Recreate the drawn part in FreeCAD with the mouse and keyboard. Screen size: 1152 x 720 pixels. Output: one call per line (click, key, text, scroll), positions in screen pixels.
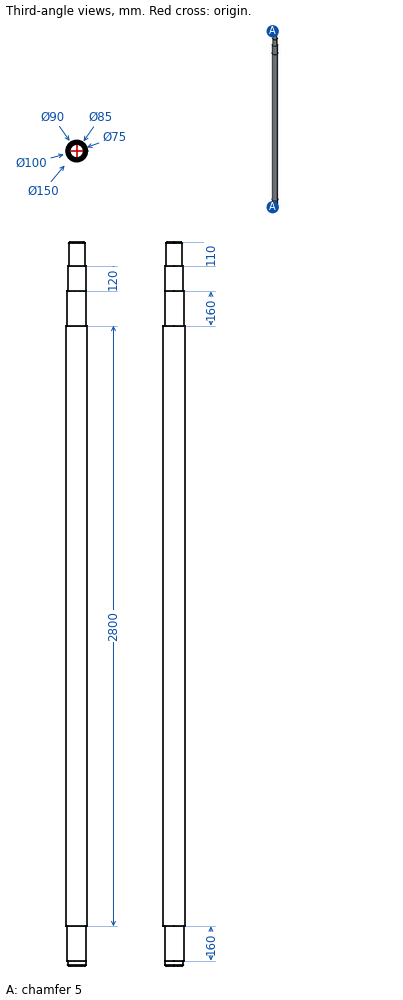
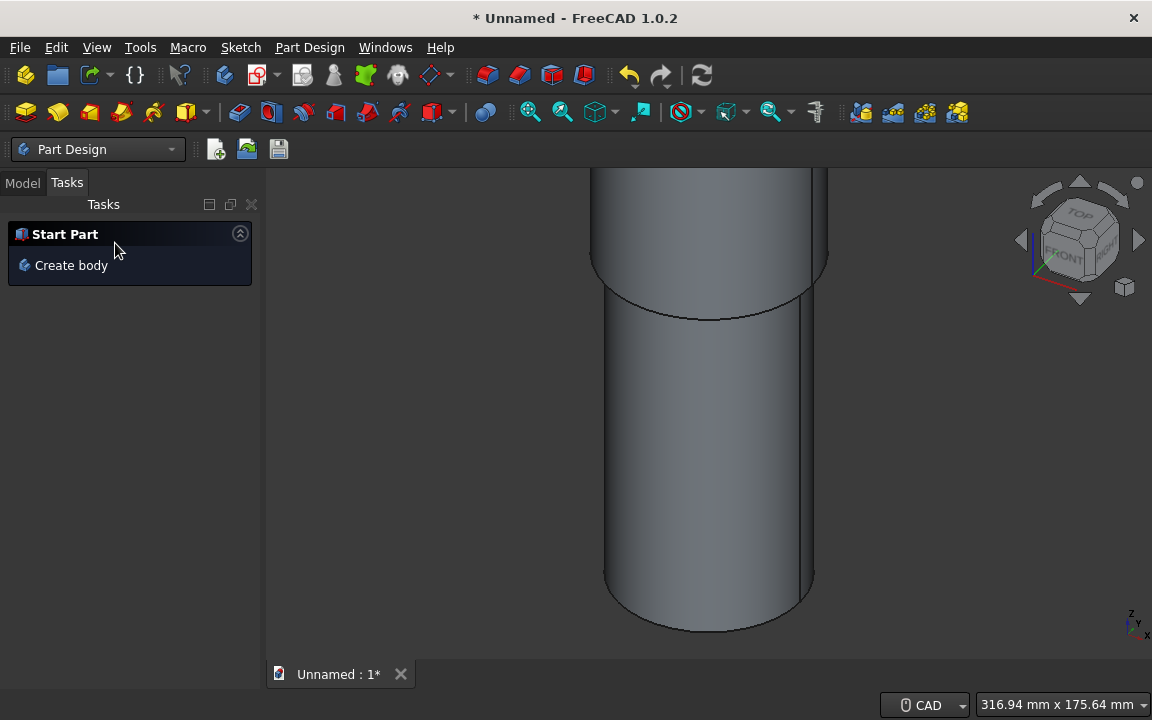
click(532, 112)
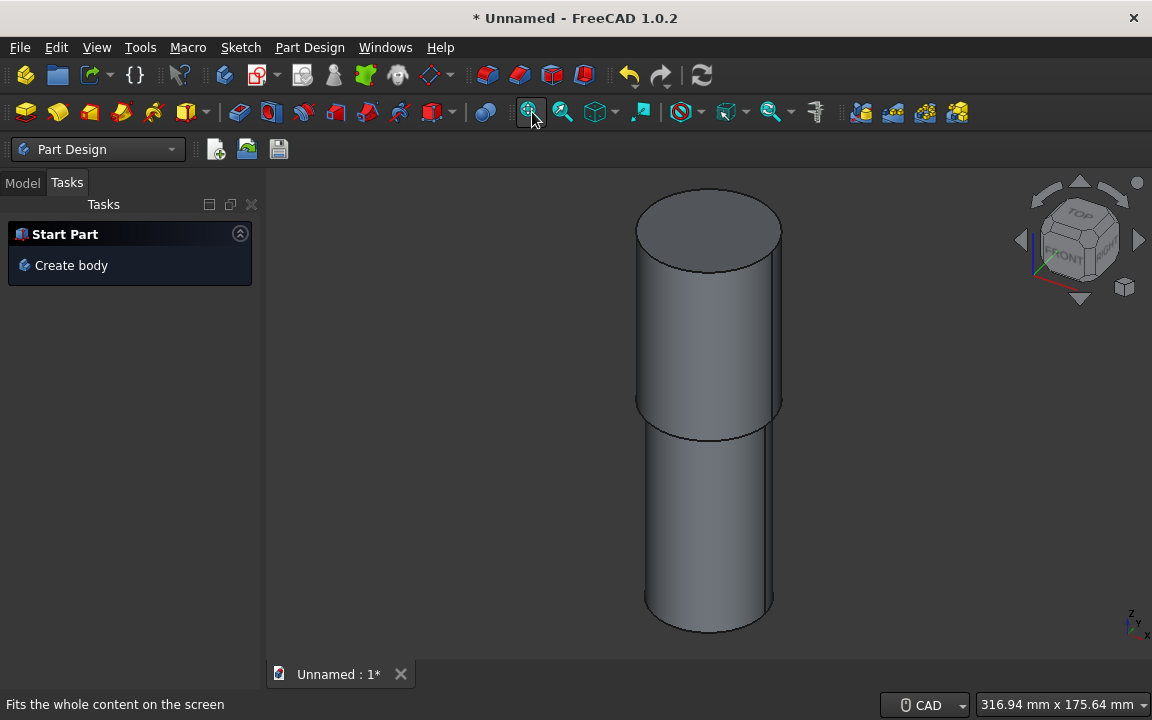
click(709, 230)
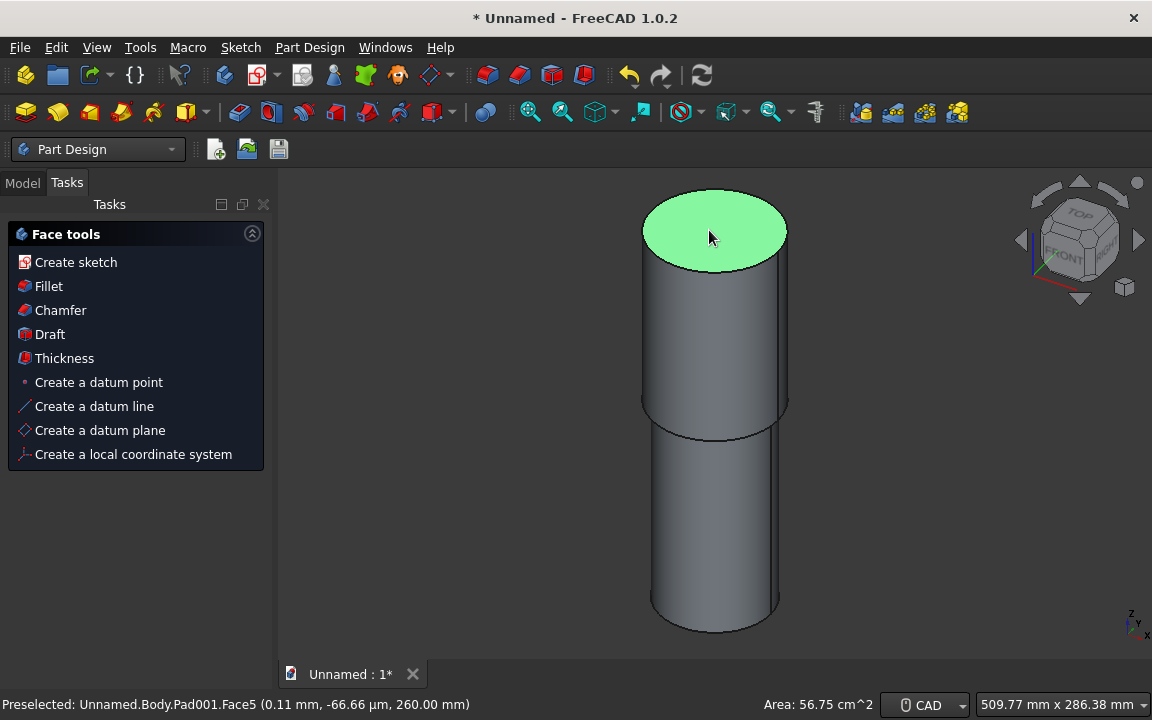
click(258, 76)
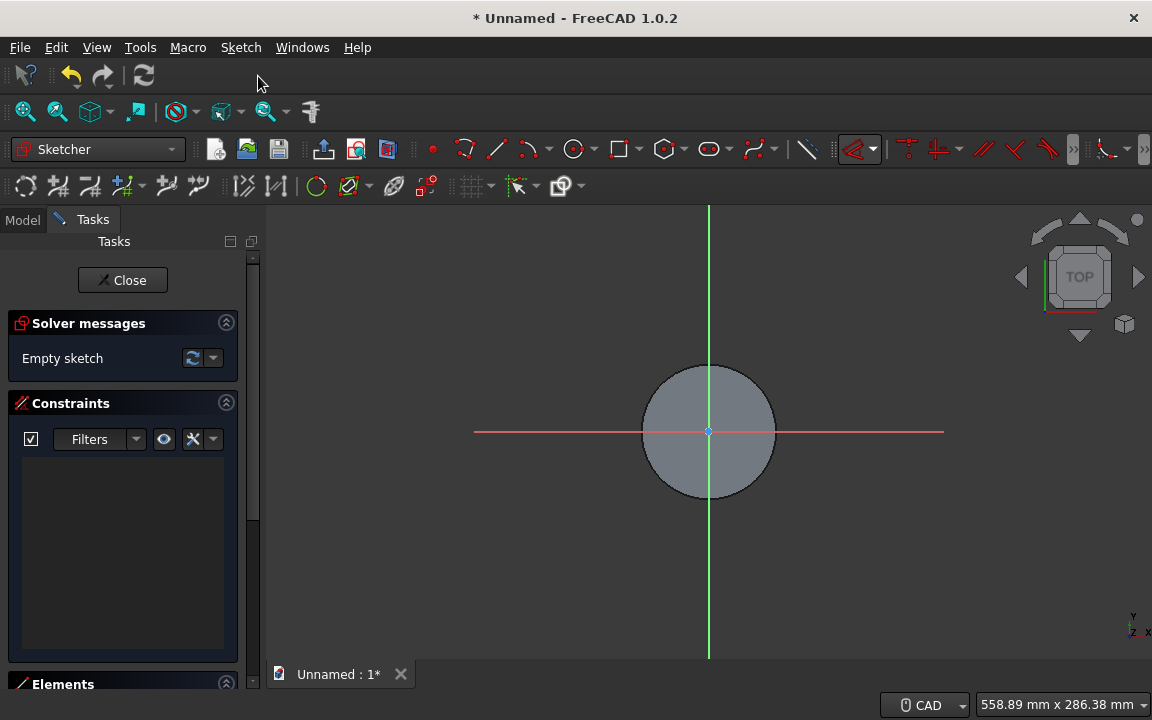
scroll(792, 432, up, 3)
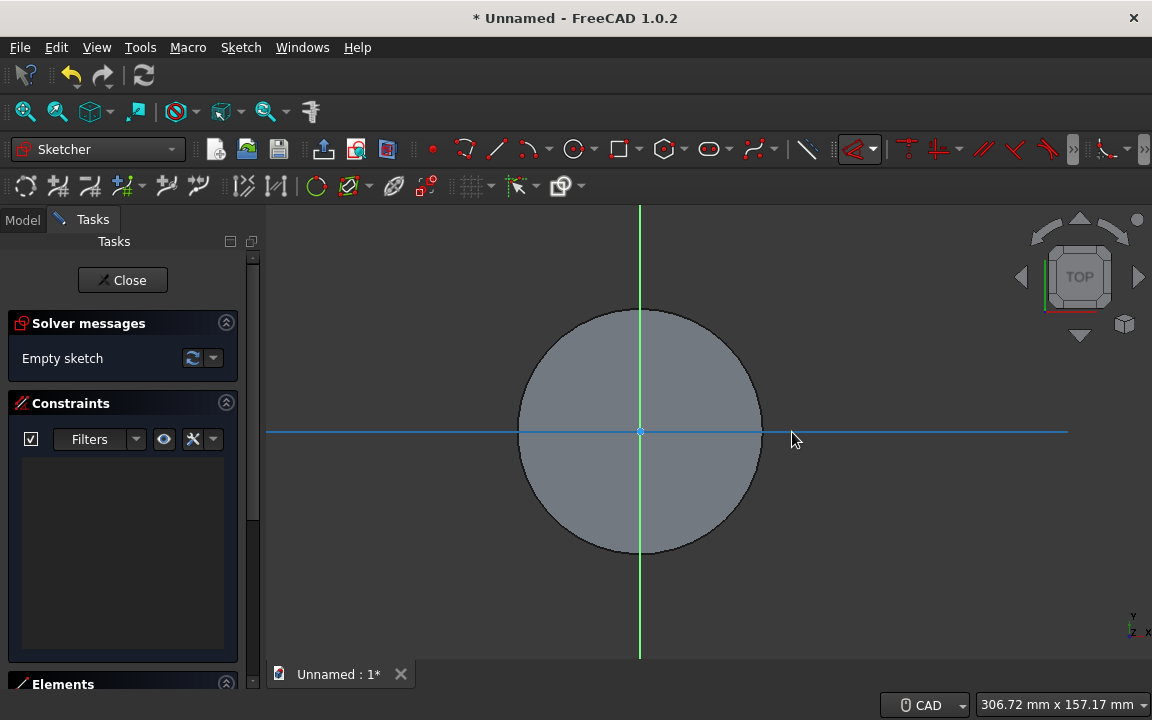
click(574, 150)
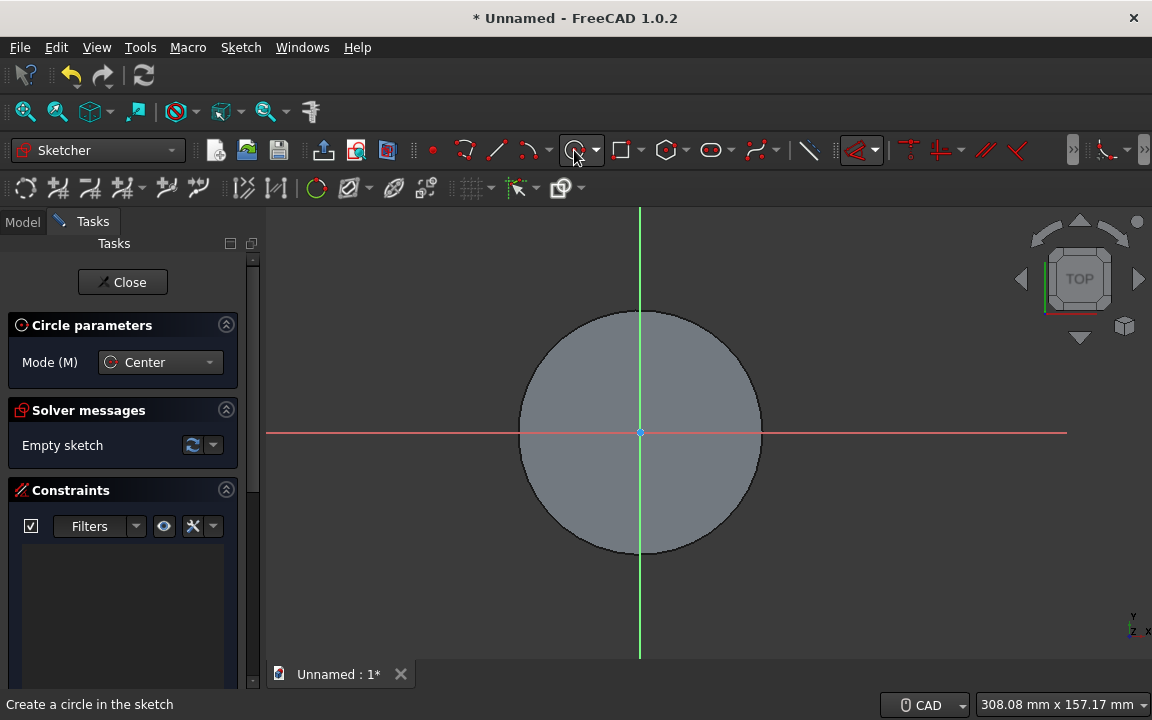
click(640, 433)
click(732, 341)
key(Escape)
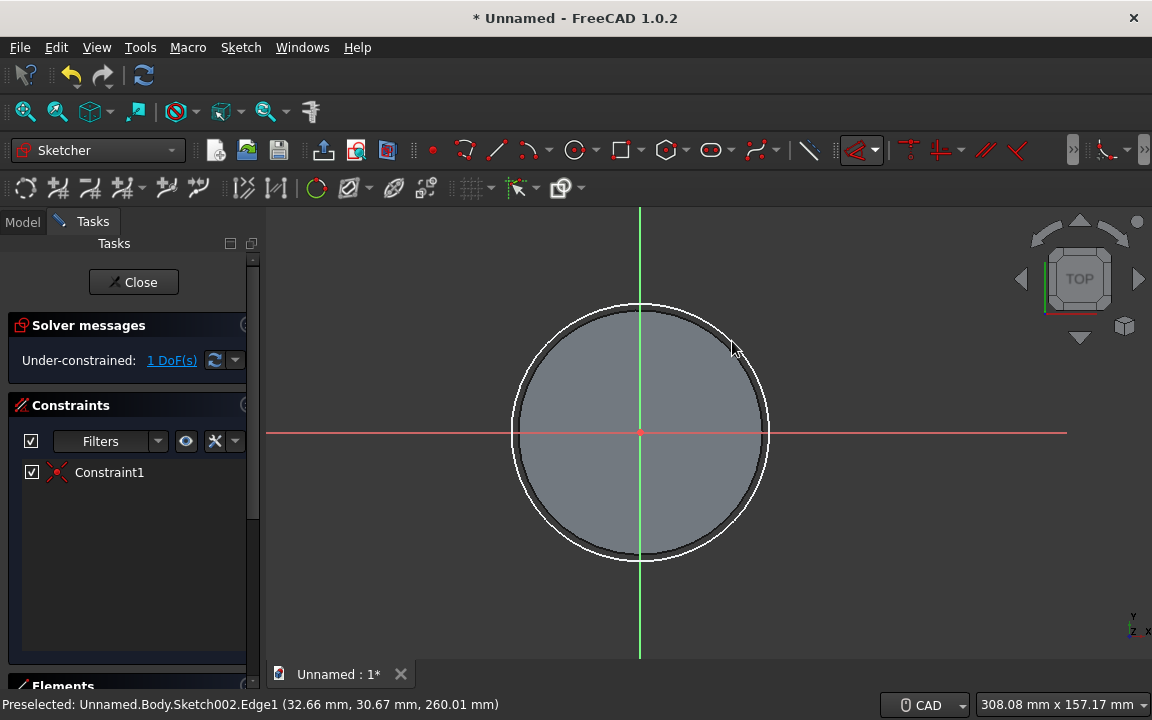
click(731, 341)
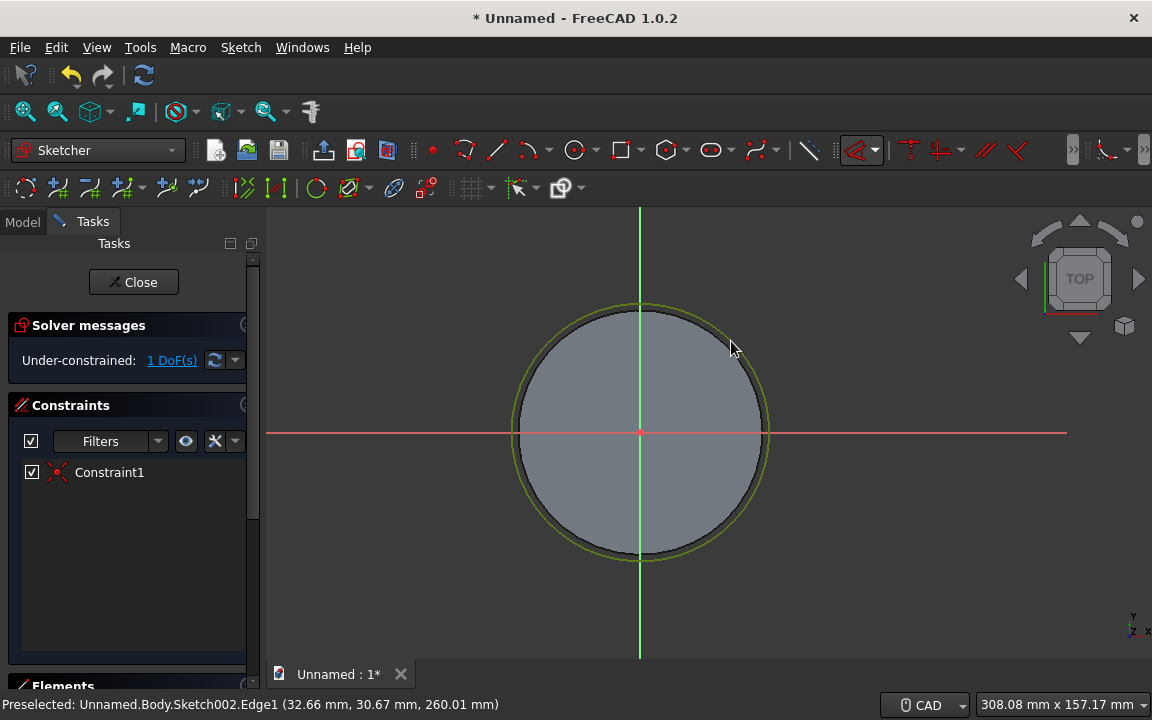
click(878, 150)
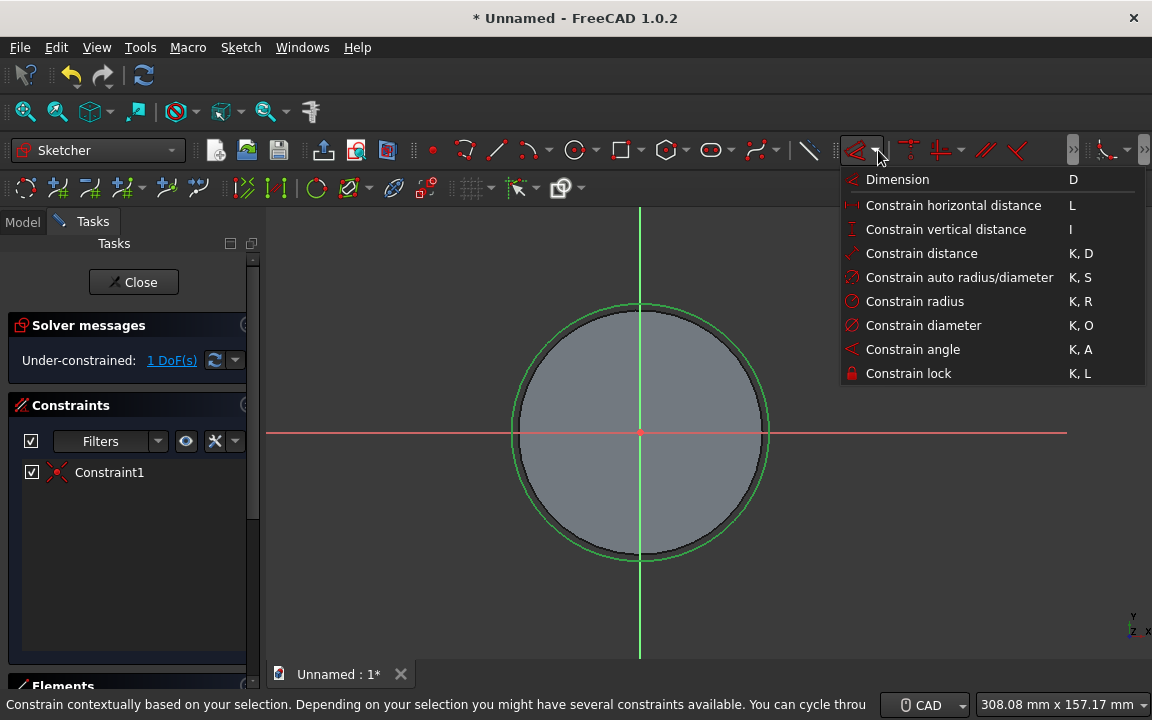
click(993, 325)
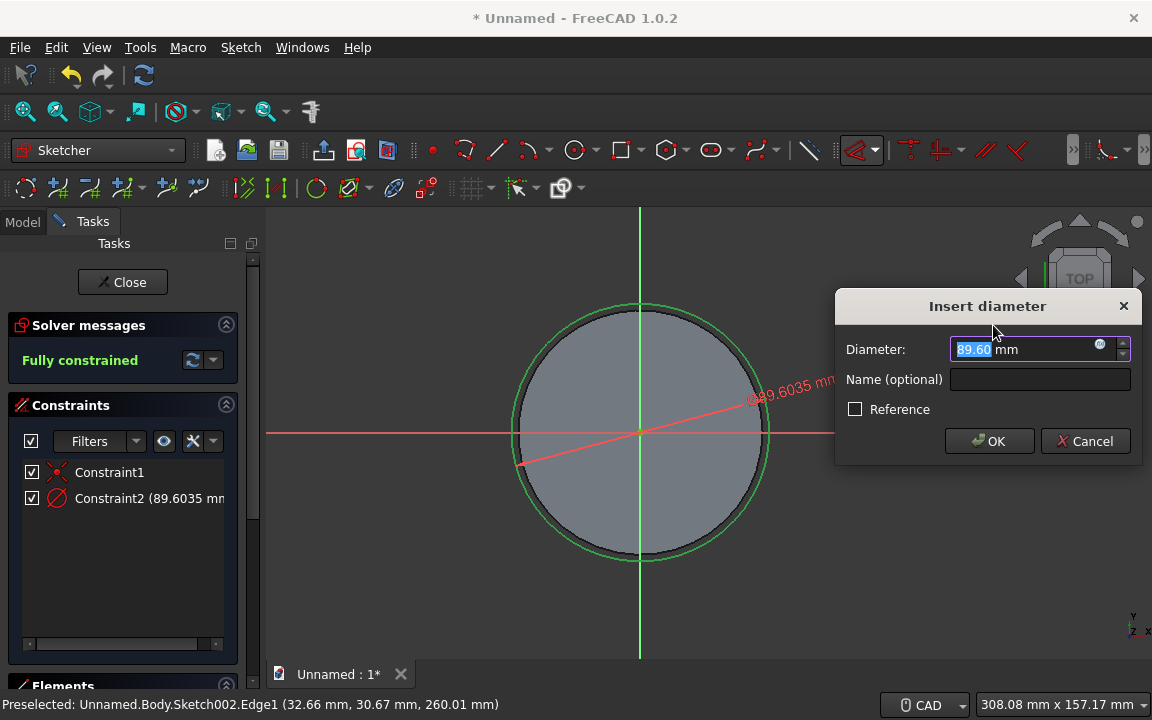
text(90)
key(Return)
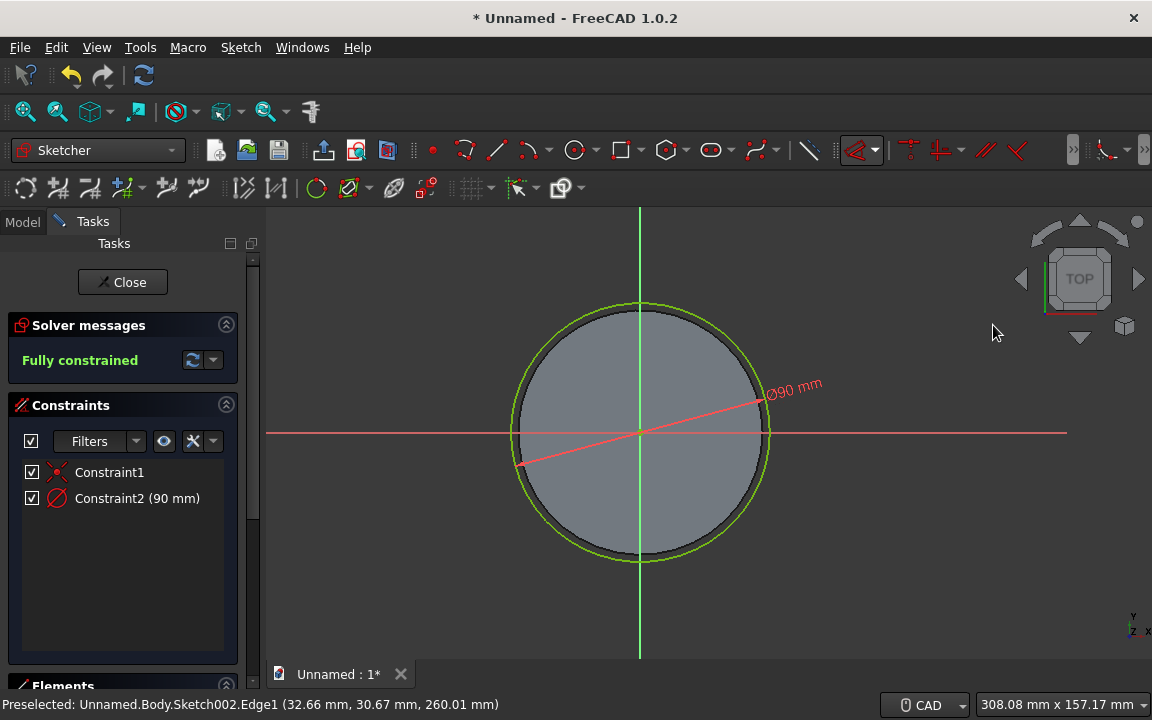
click(123, 282)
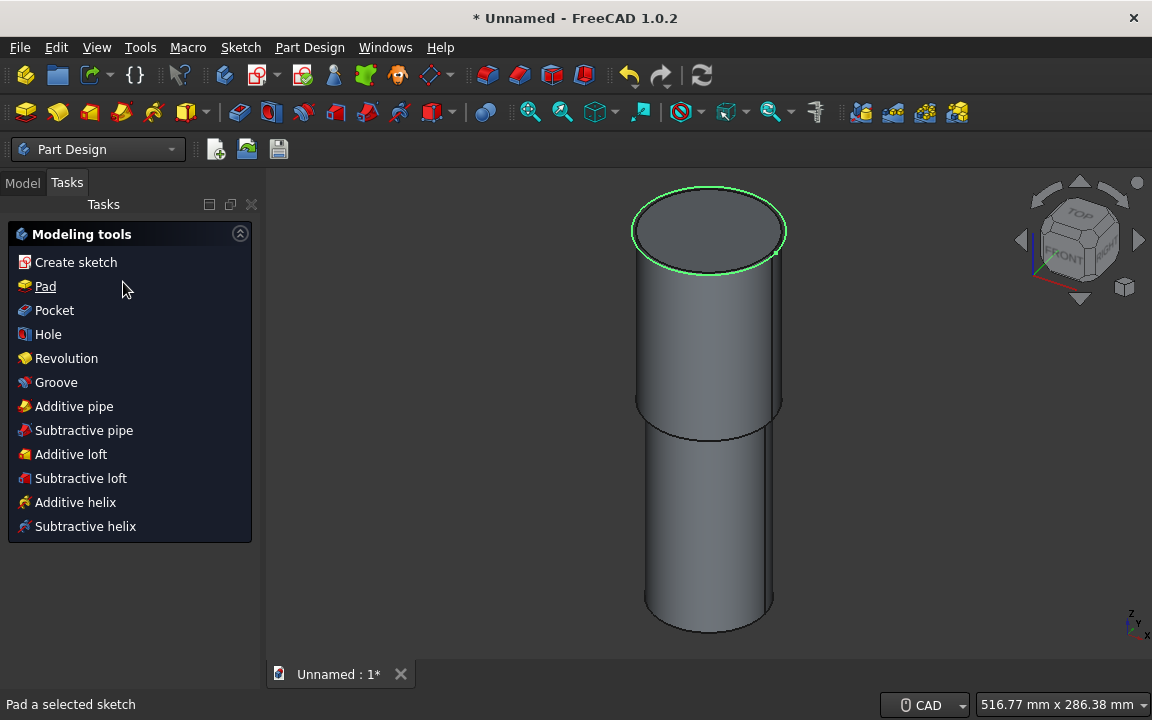
click(26, 112)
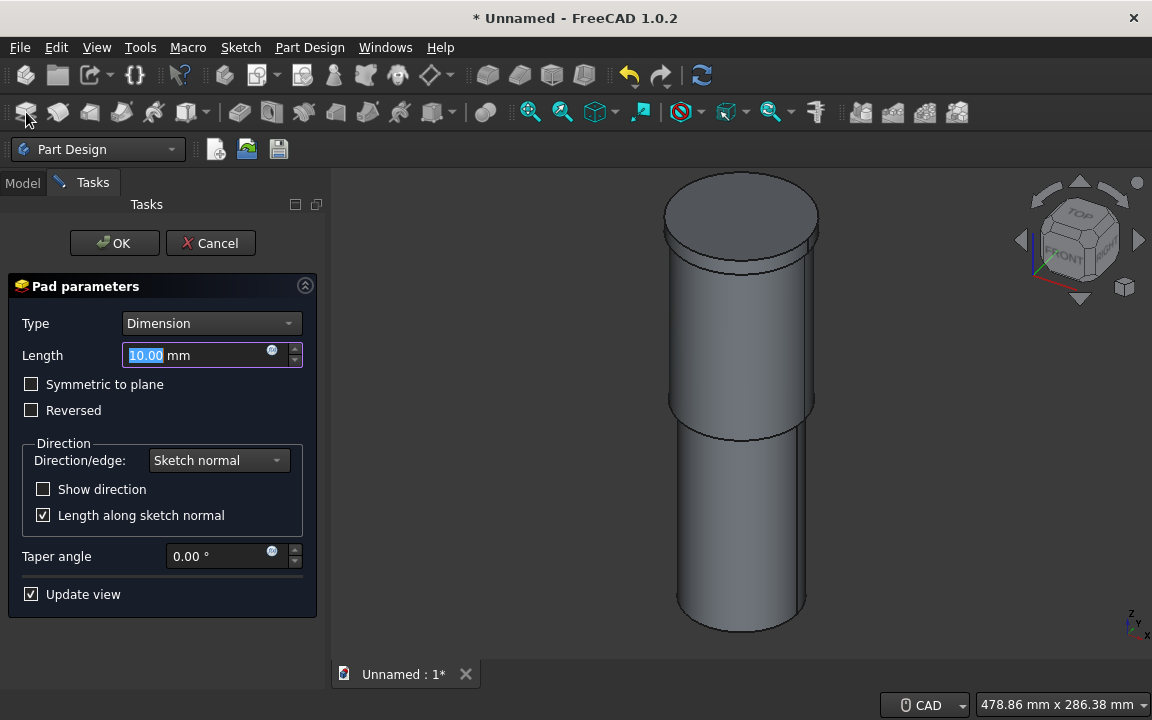
text(160)
key(Tab)